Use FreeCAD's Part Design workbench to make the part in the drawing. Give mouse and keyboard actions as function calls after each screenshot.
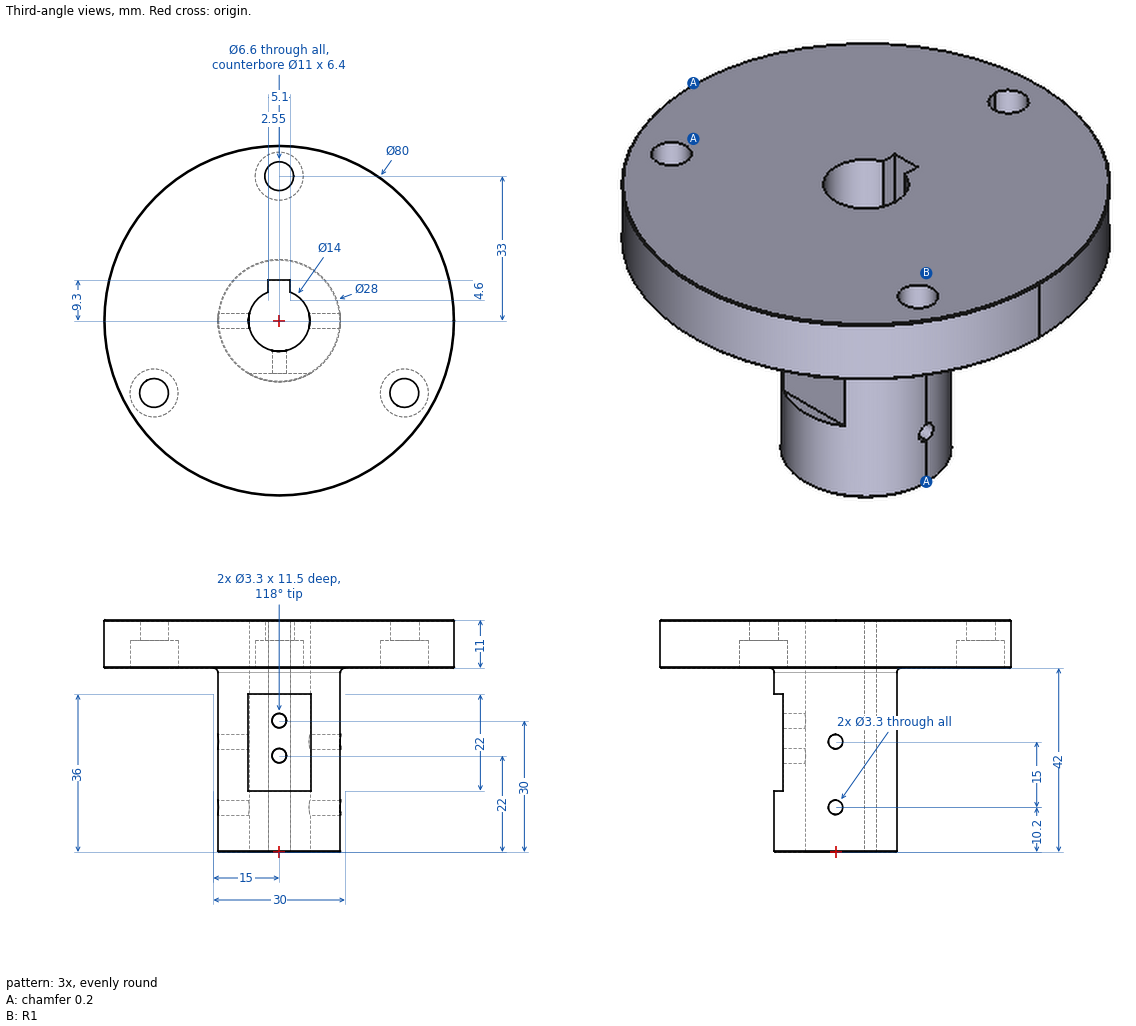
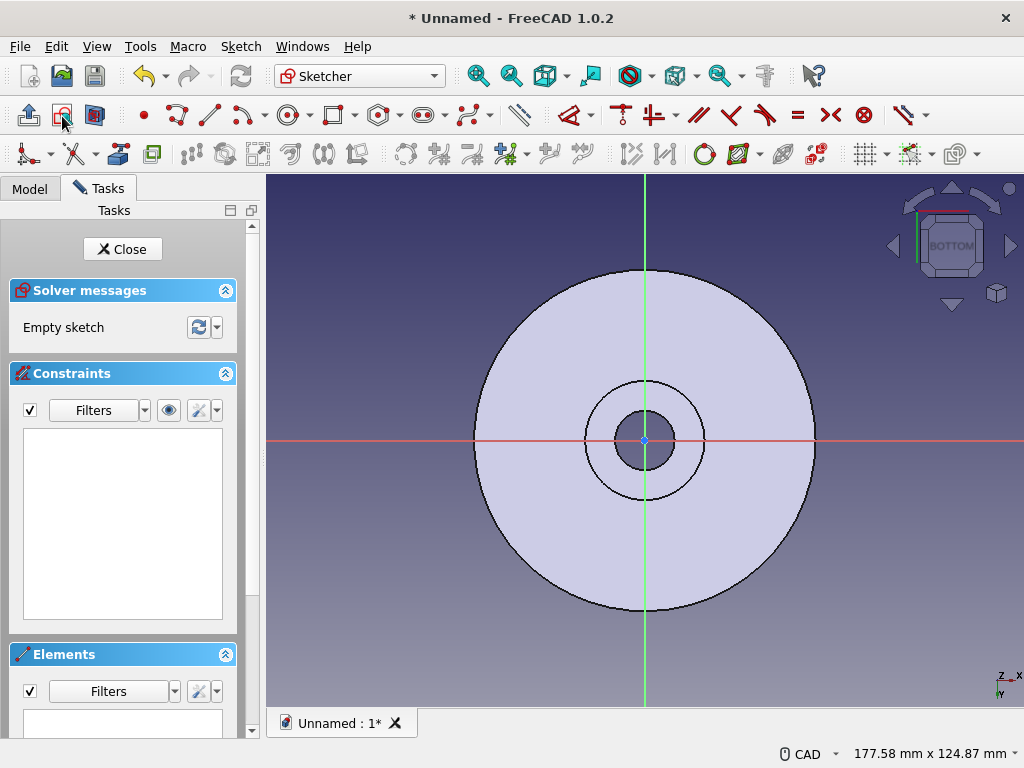
scroll(652, 595, up, 12)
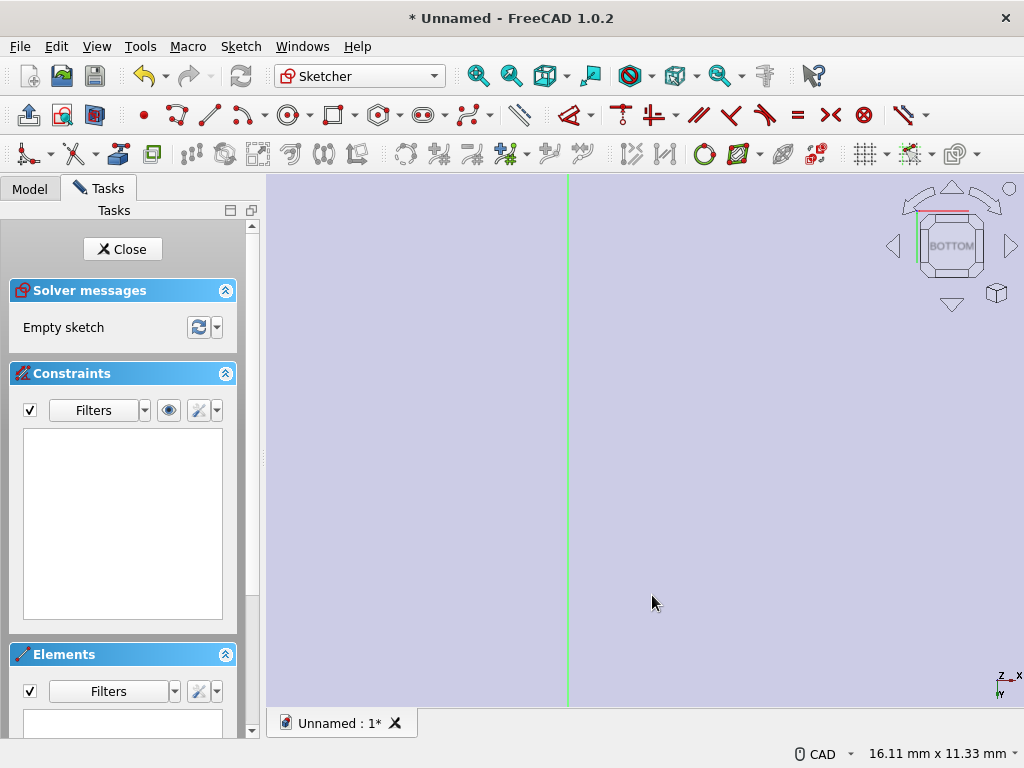
key(g)
key(c)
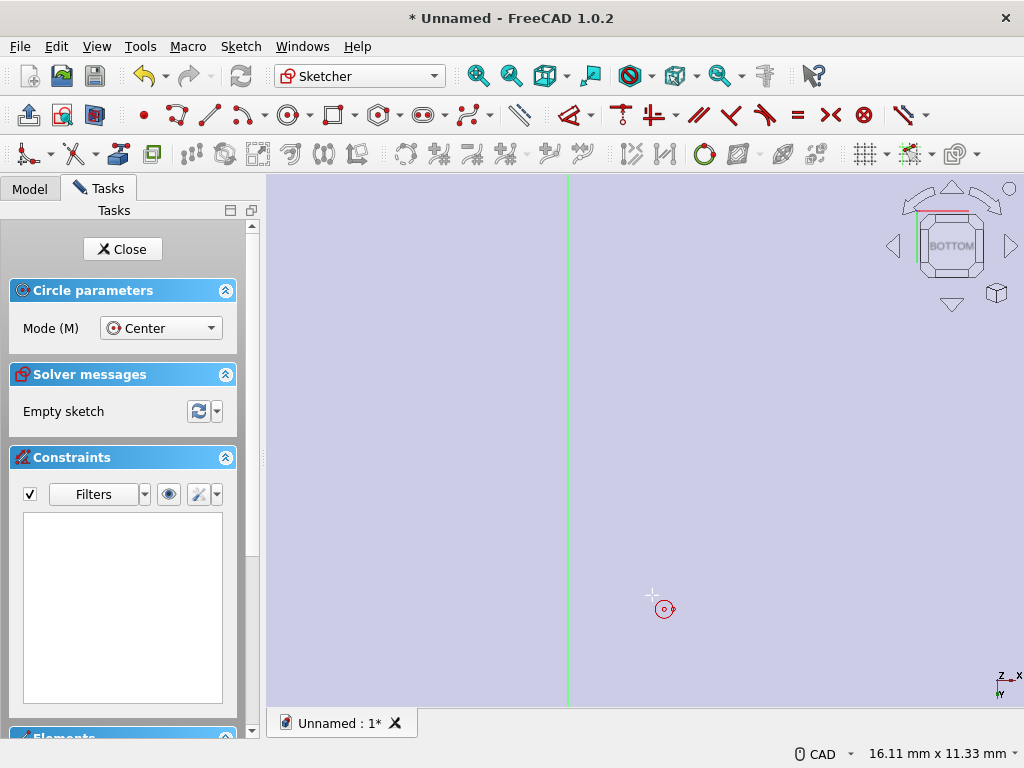
click(568, 437)
move(678, 327)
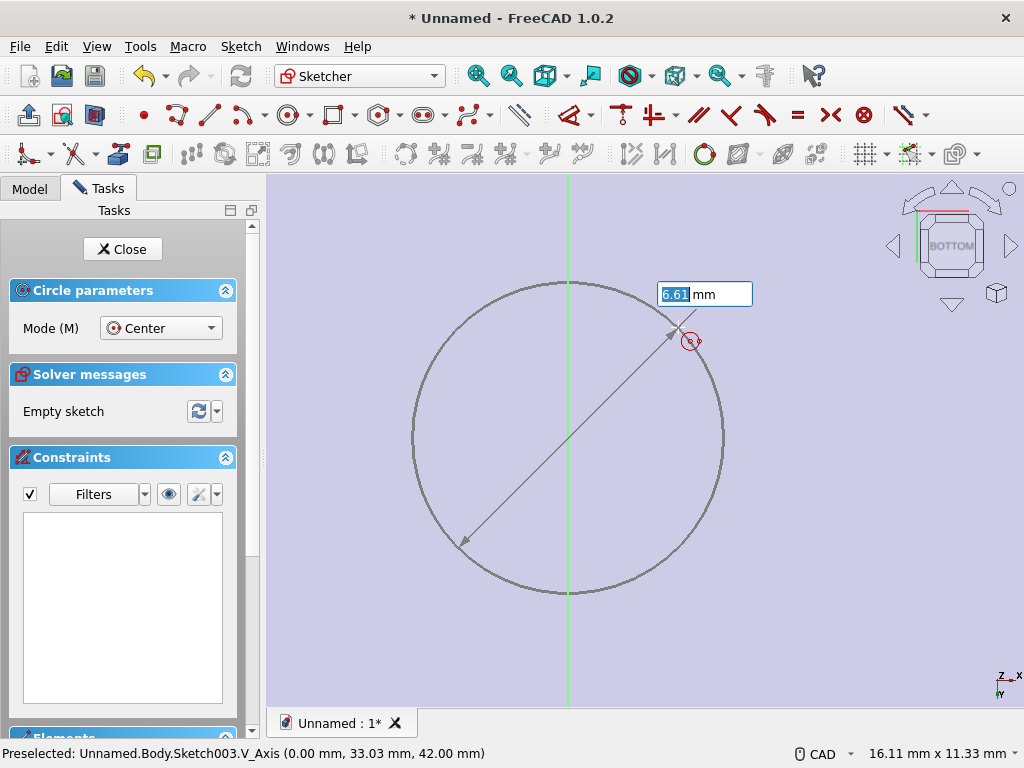
text(6.6)
key(Return)
key(Escape)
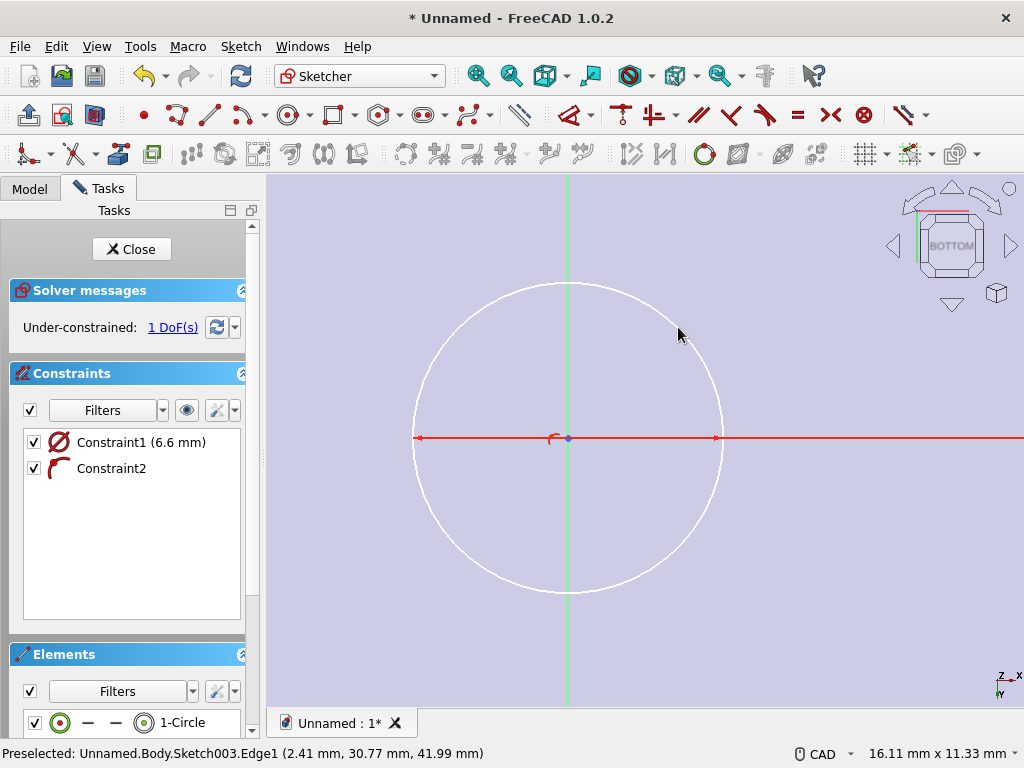
click(568, 438)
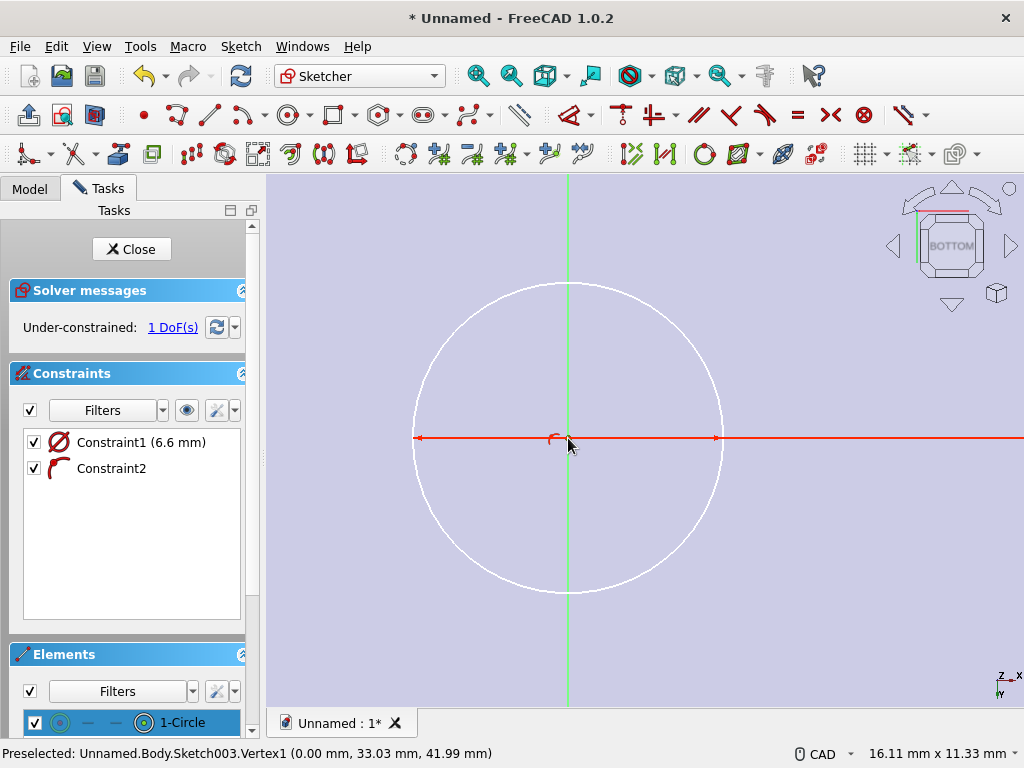
key(i)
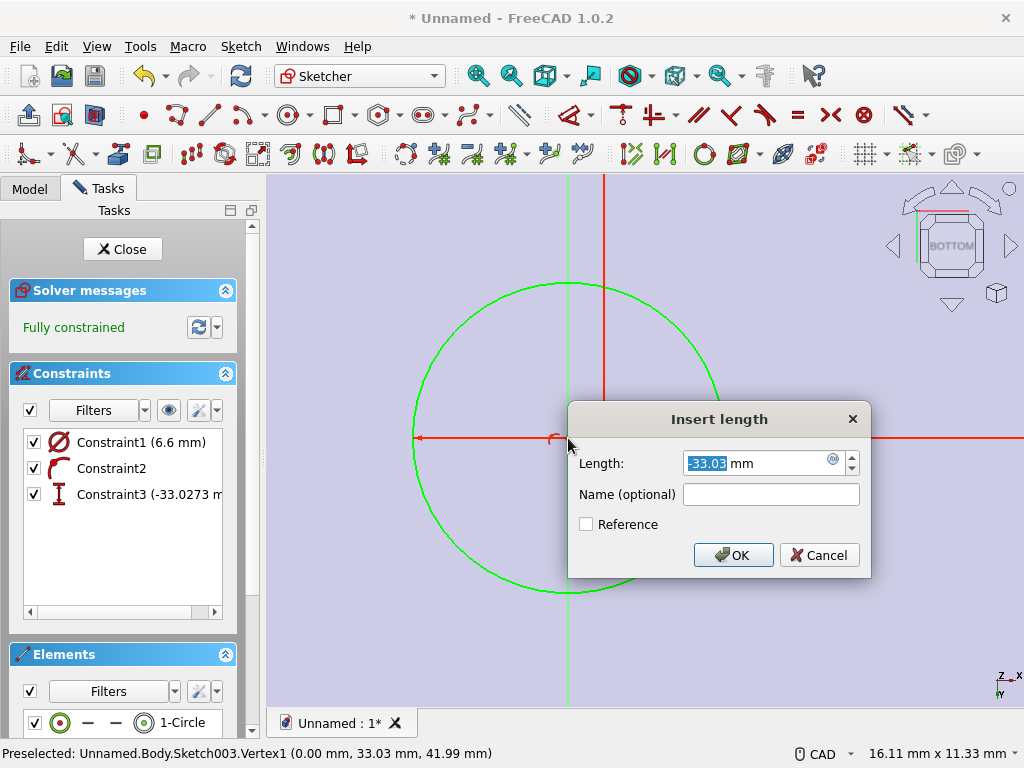
text(-33)
key(Return)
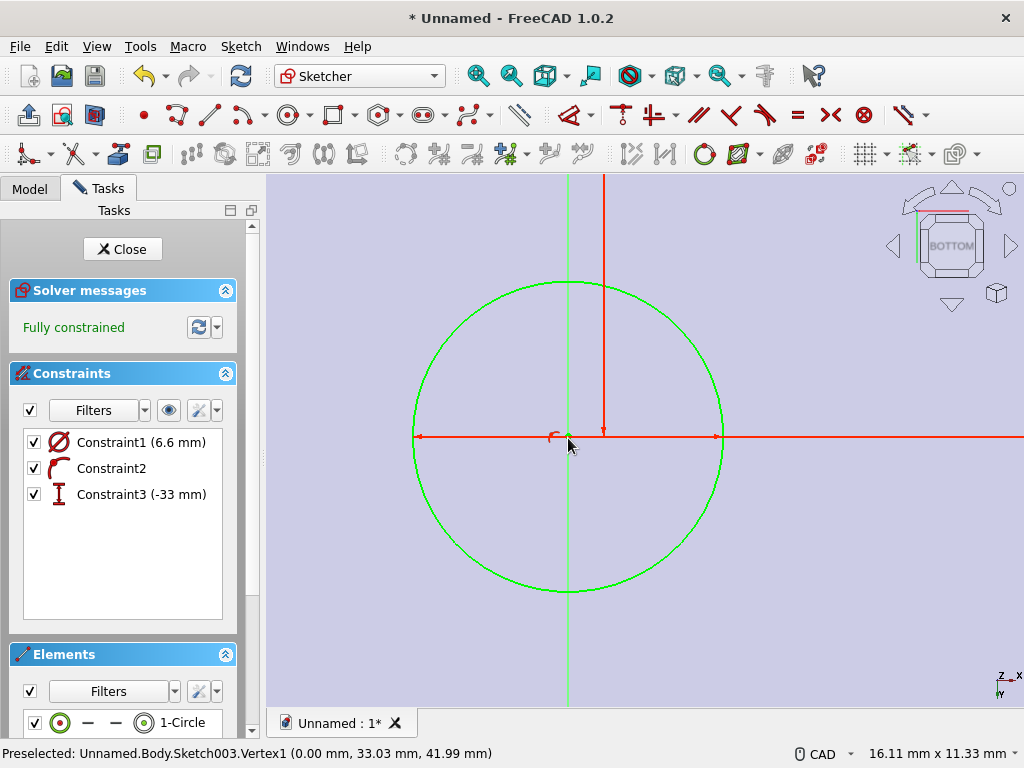
click(123, 249)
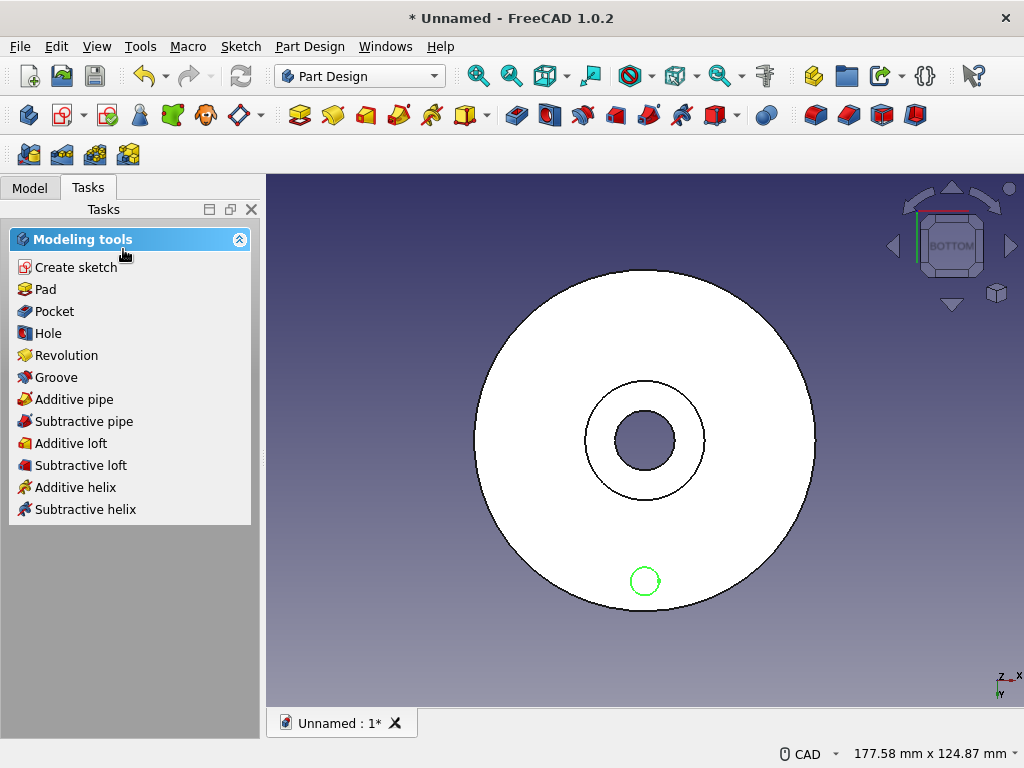
click(550, 116)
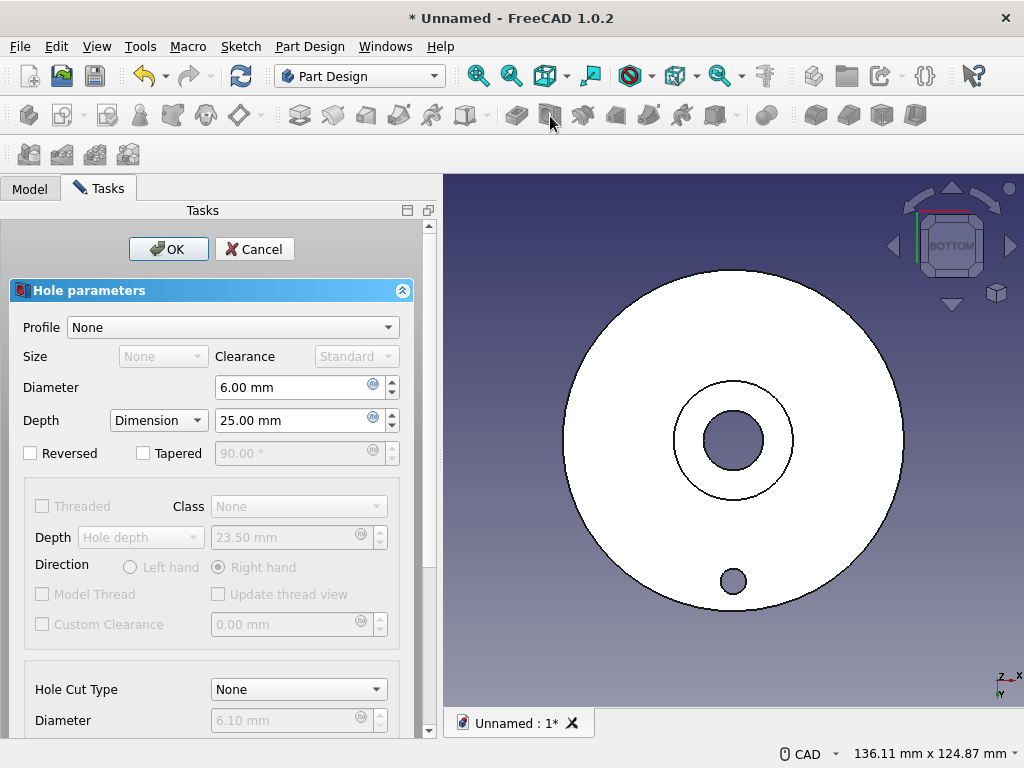
triple_click(300, 388)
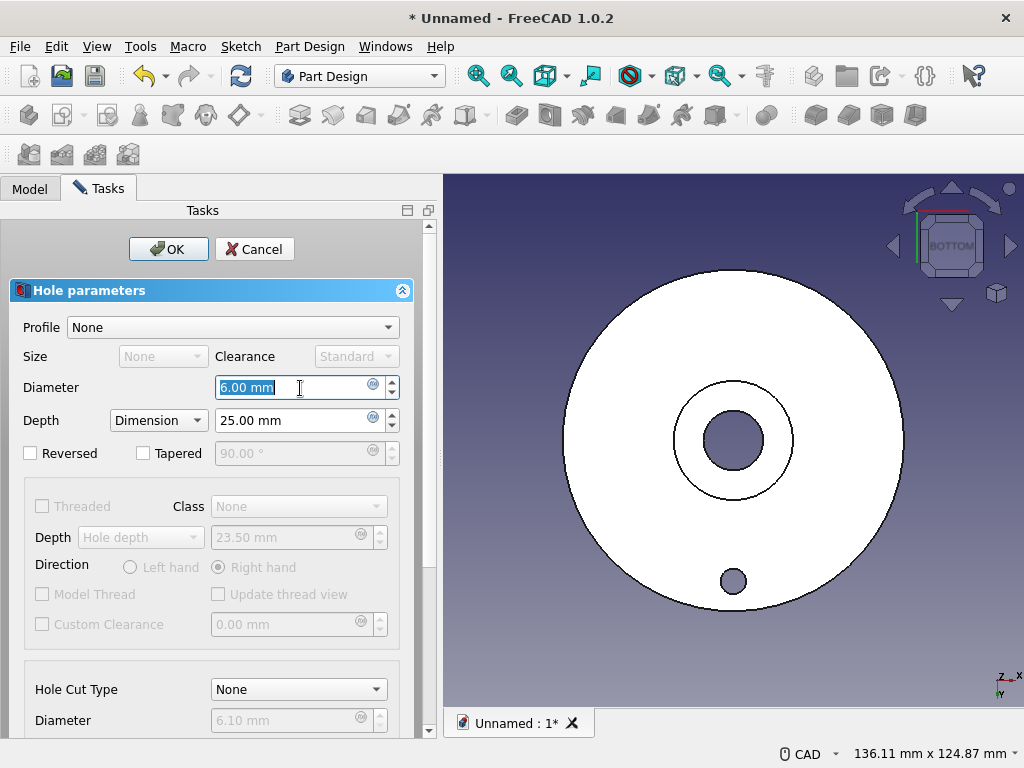
text(6.6)
key(Tab)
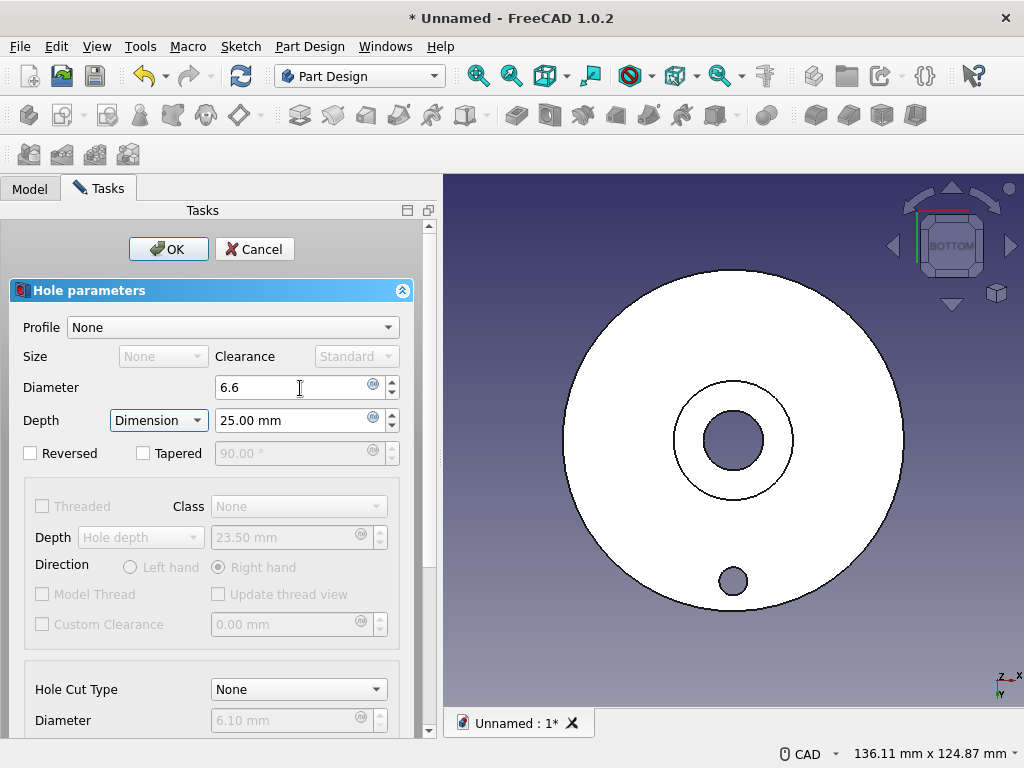
click(160, 420)